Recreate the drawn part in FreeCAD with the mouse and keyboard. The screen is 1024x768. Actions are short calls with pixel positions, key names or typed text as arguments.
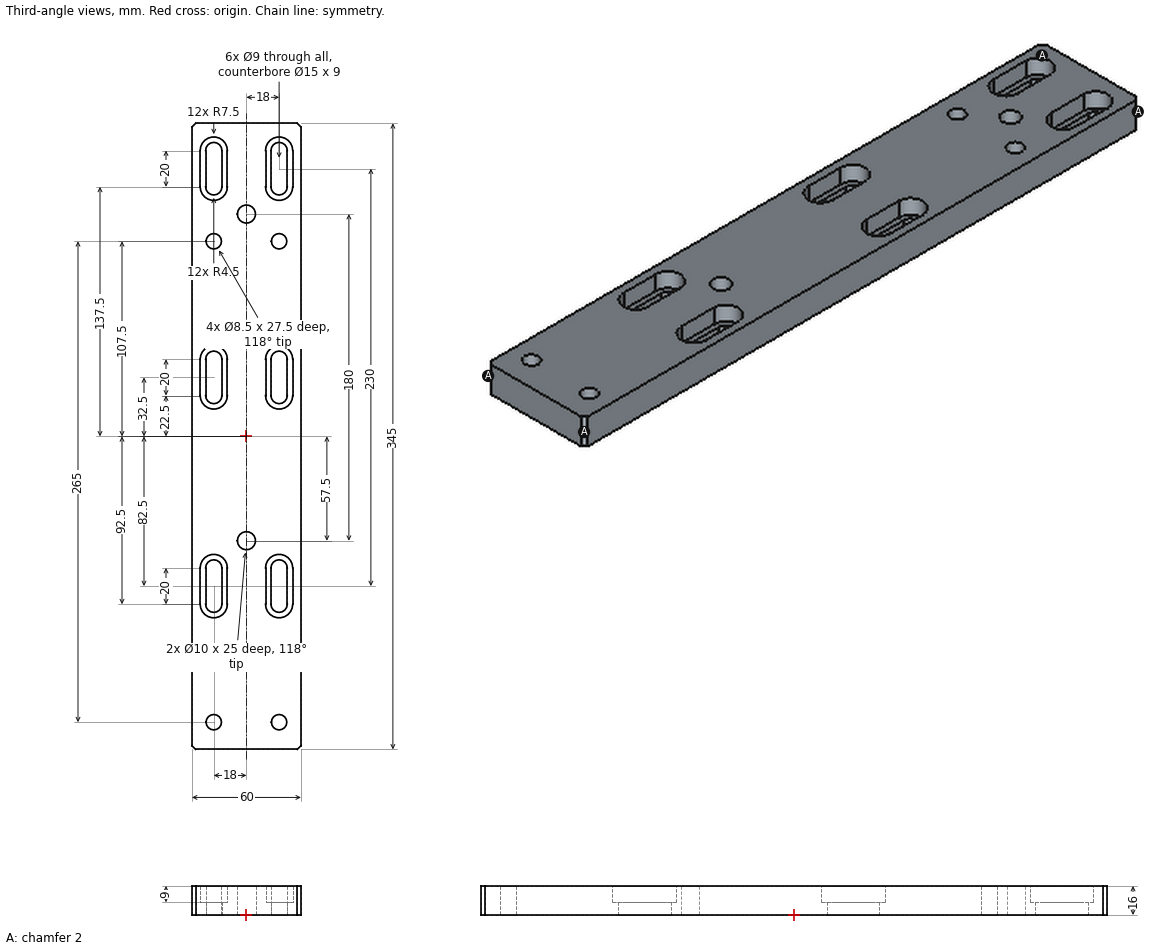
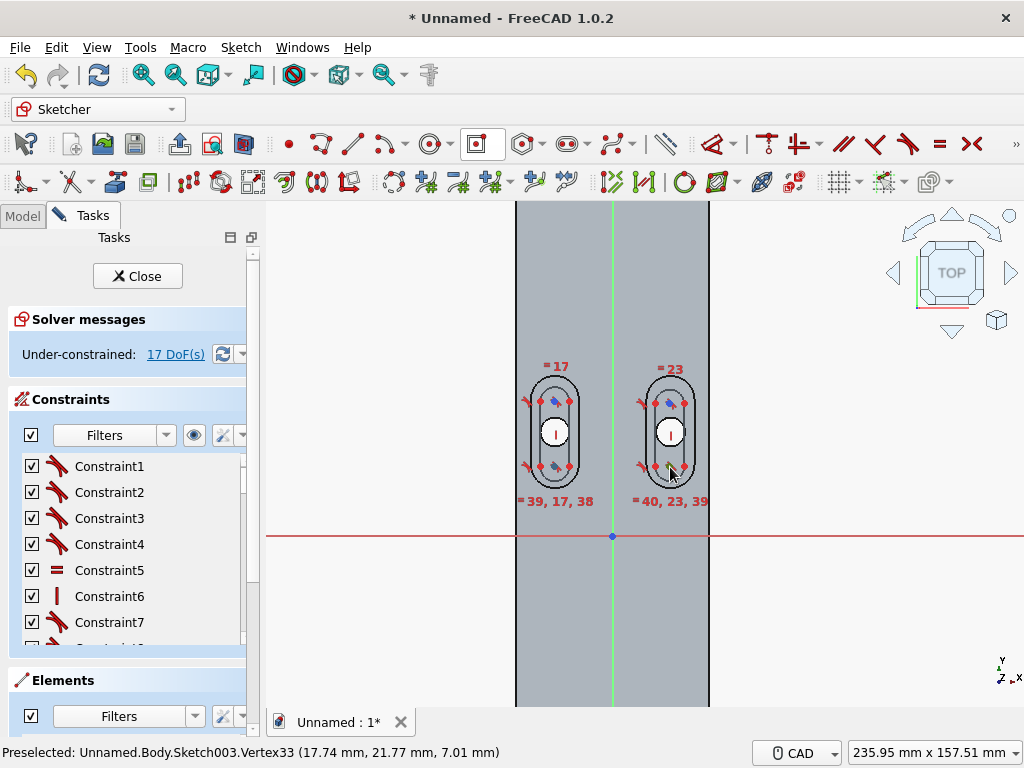
click(613, 647)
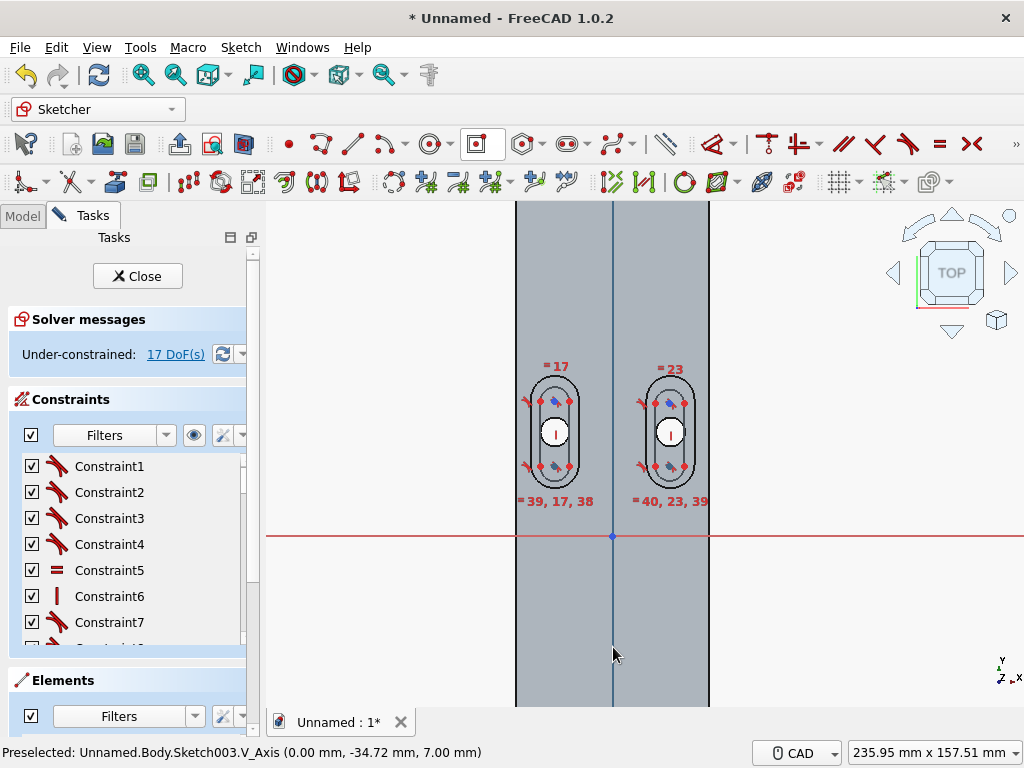
key(s)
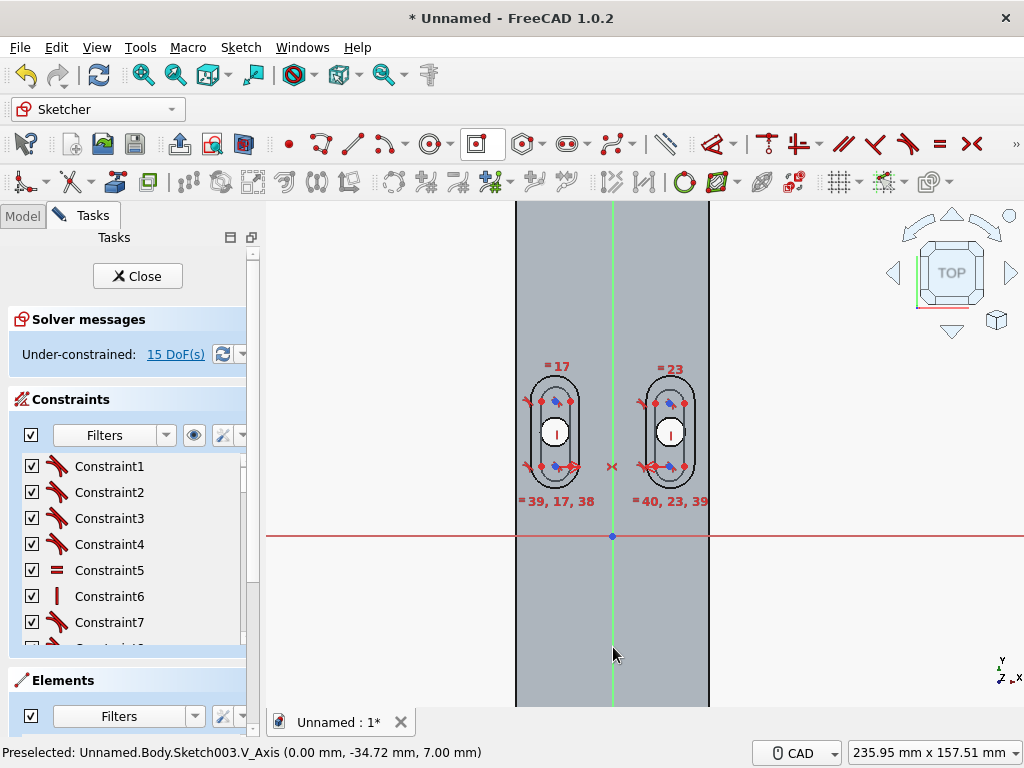
scroll(555, 467, down, 5)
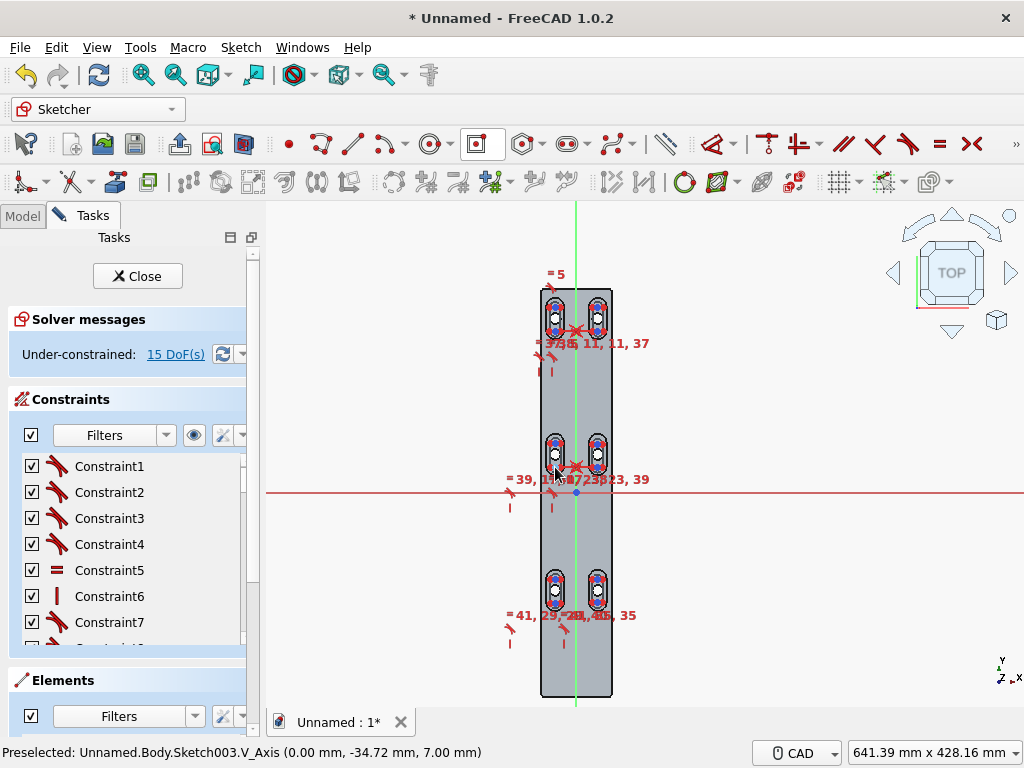
scroll(555, 603, up, 5)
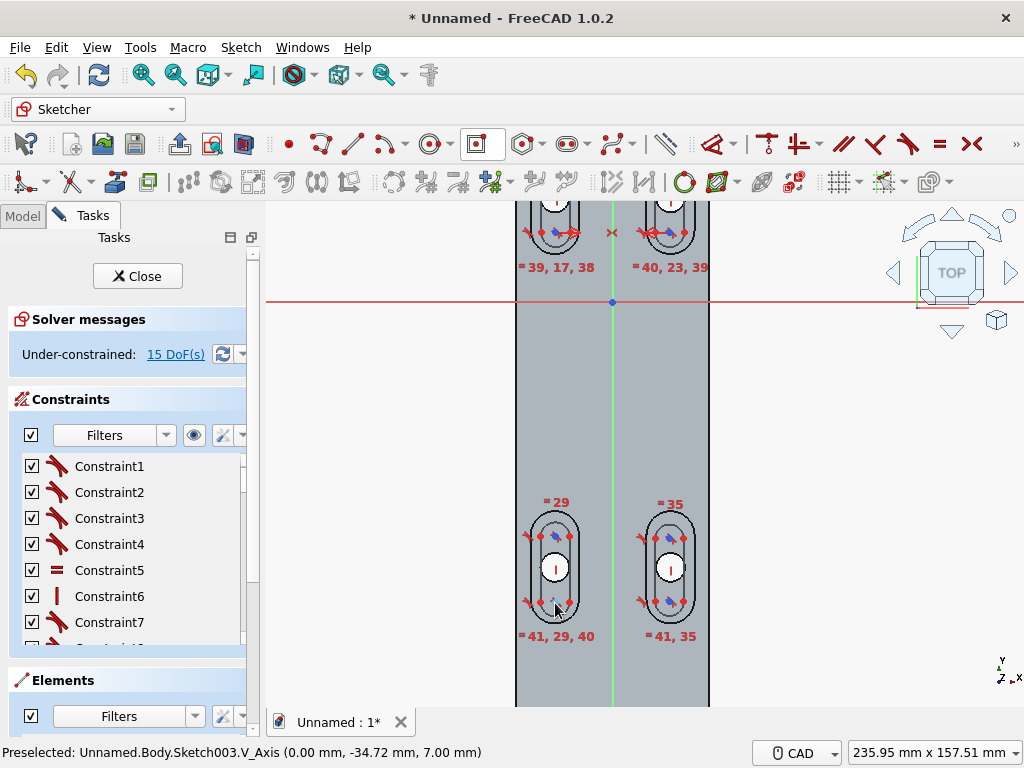
click(555, 602)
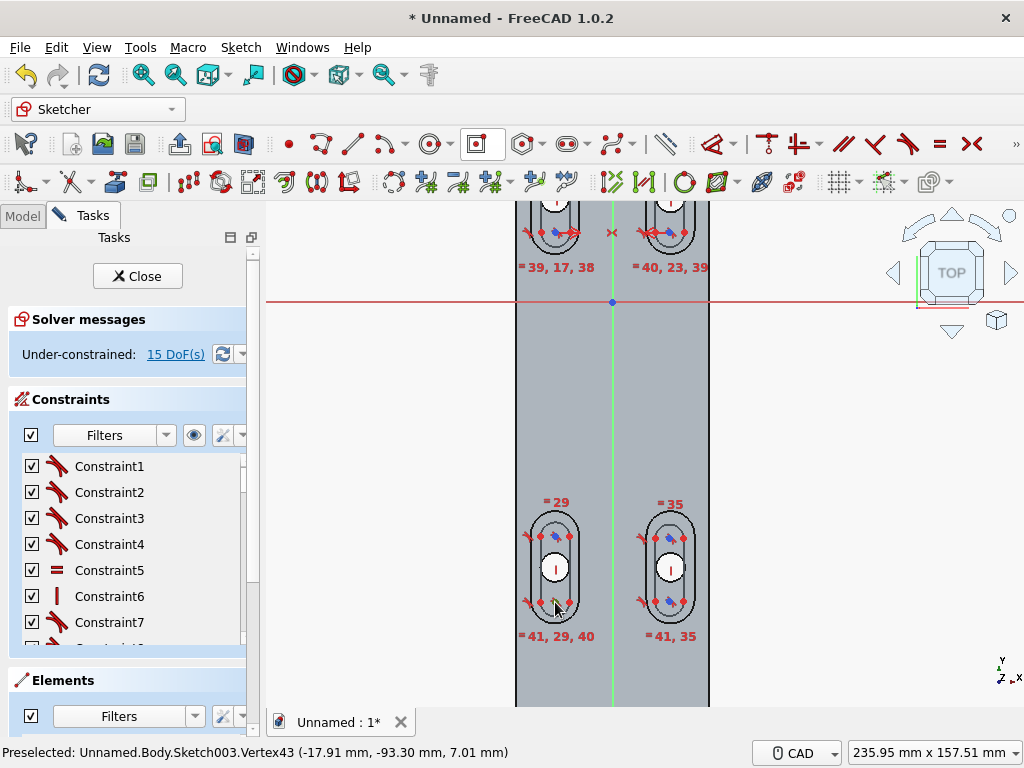
click(670, 601)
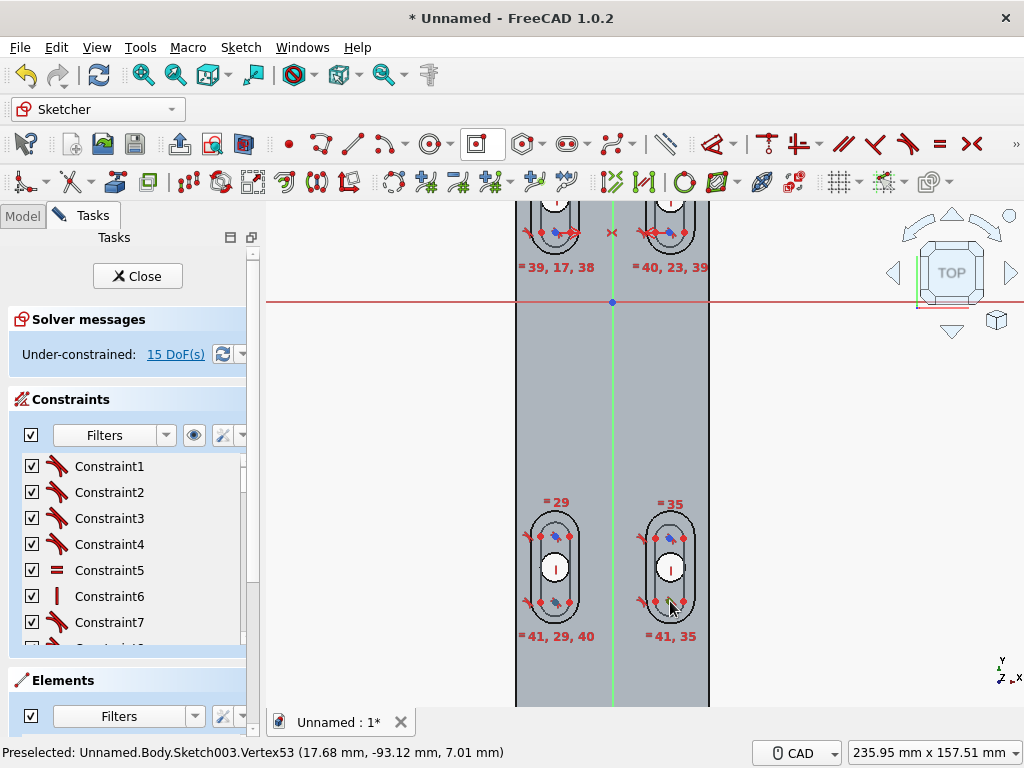
click(613, 647)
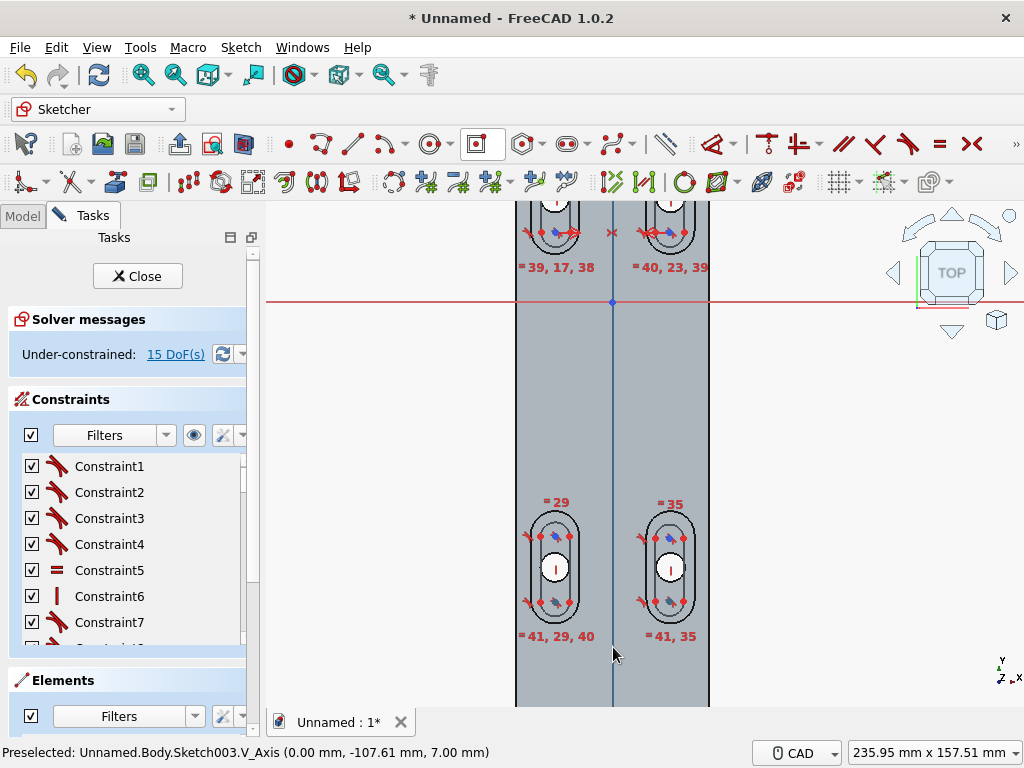
key(s)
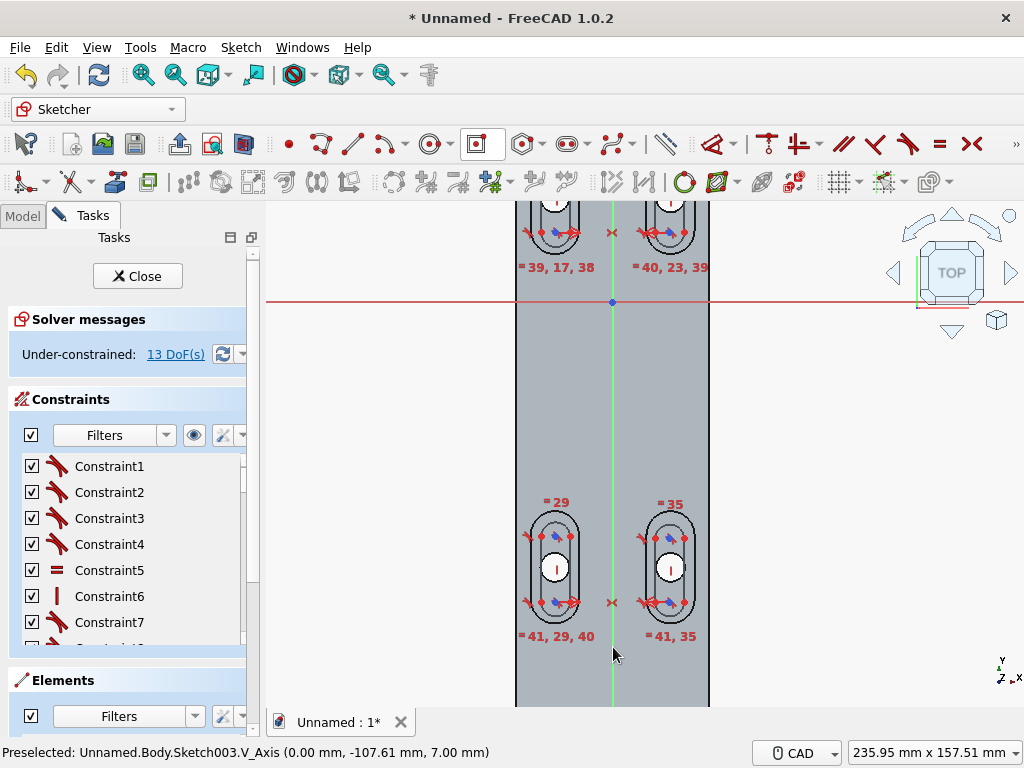
key(d)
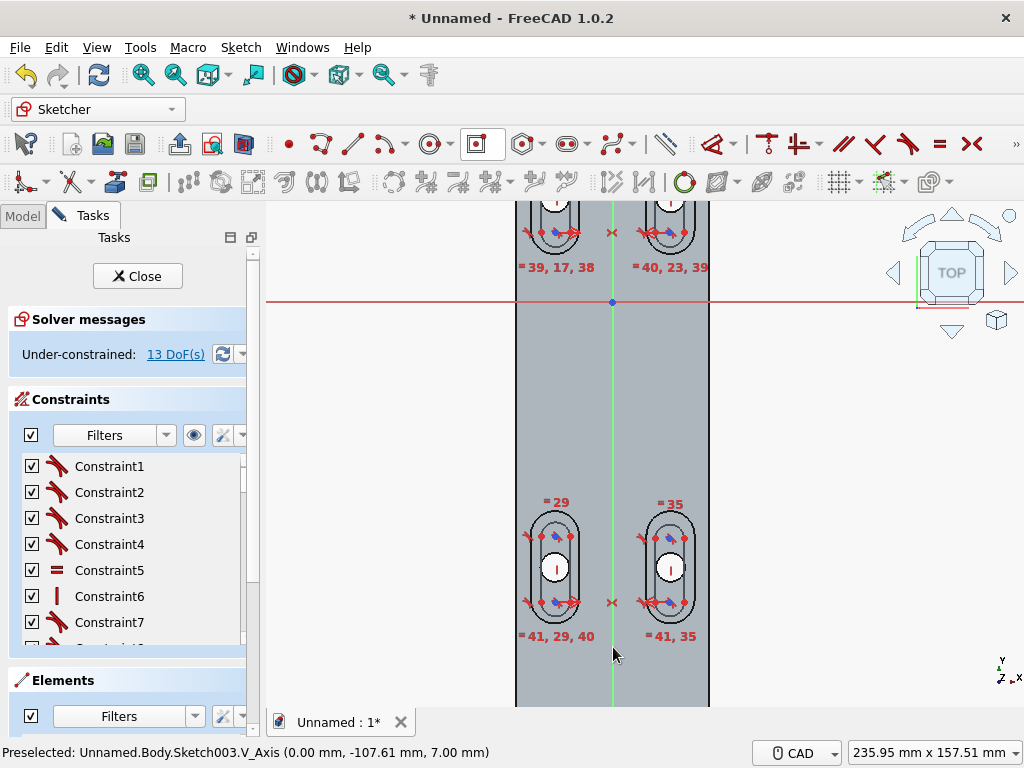
scroll(555, 603, down, 5)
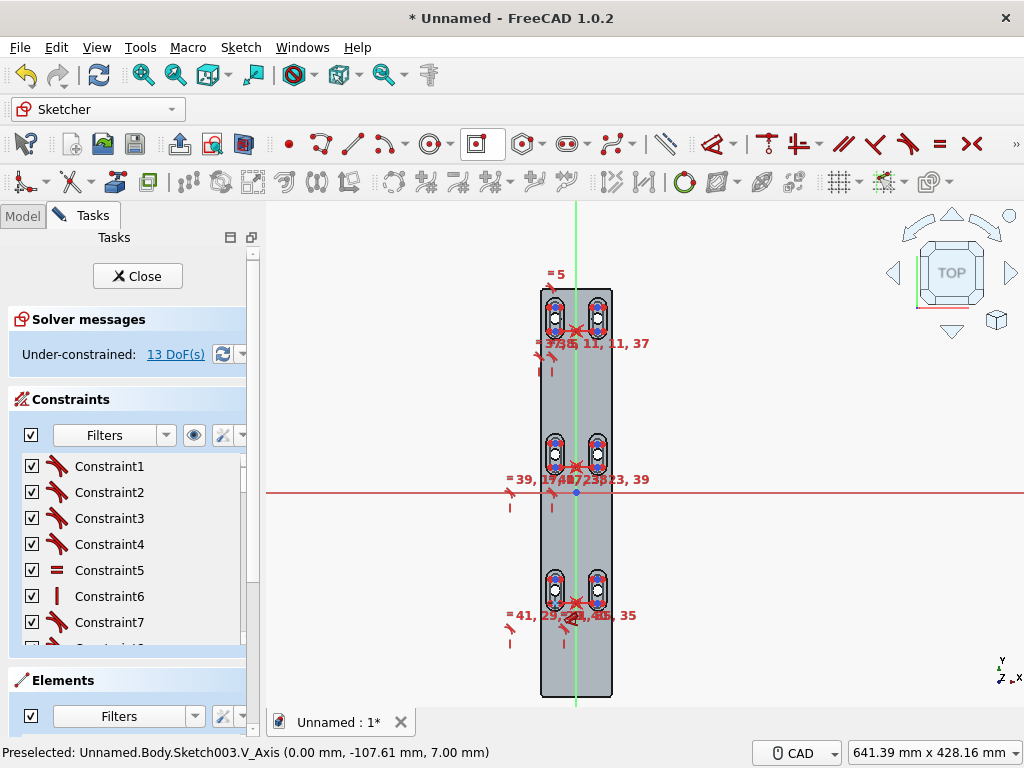
scroll(552, 336, up, 11)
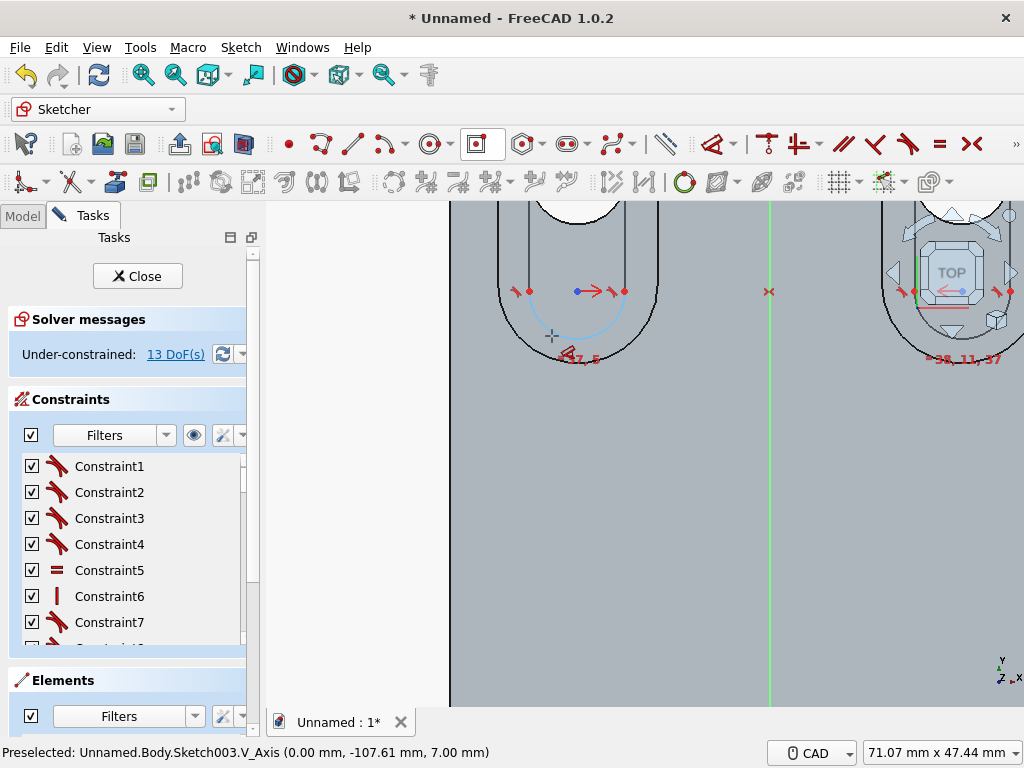
click(549, 330)
click(530, 356)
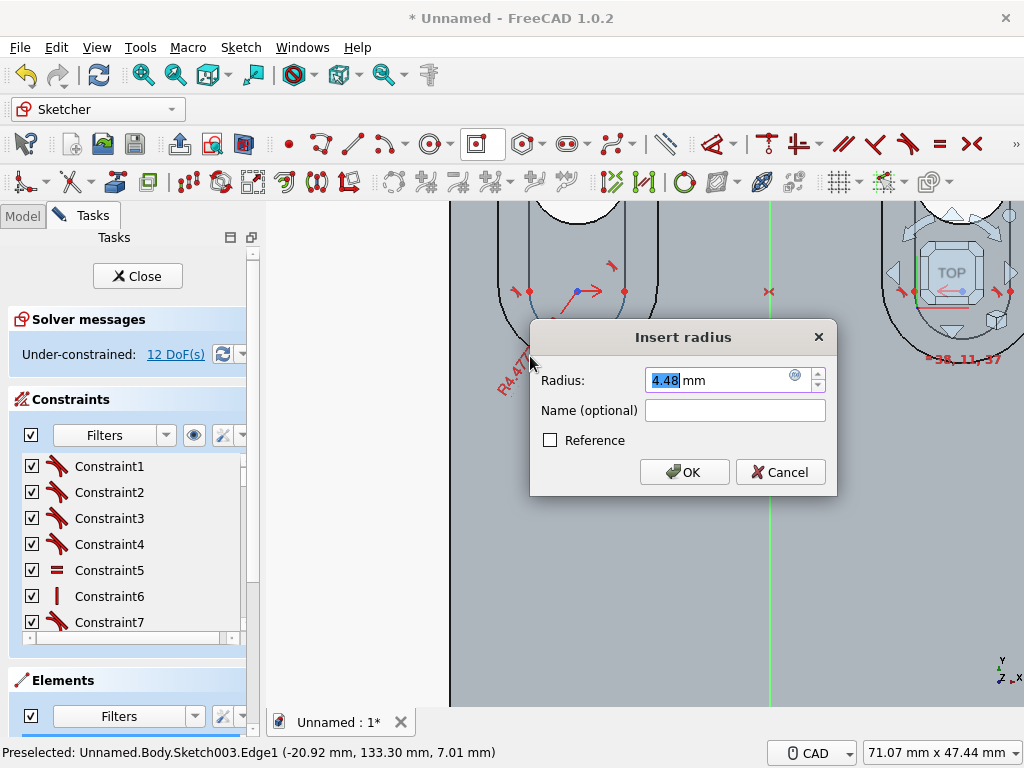
text(4.5)
key(Return)